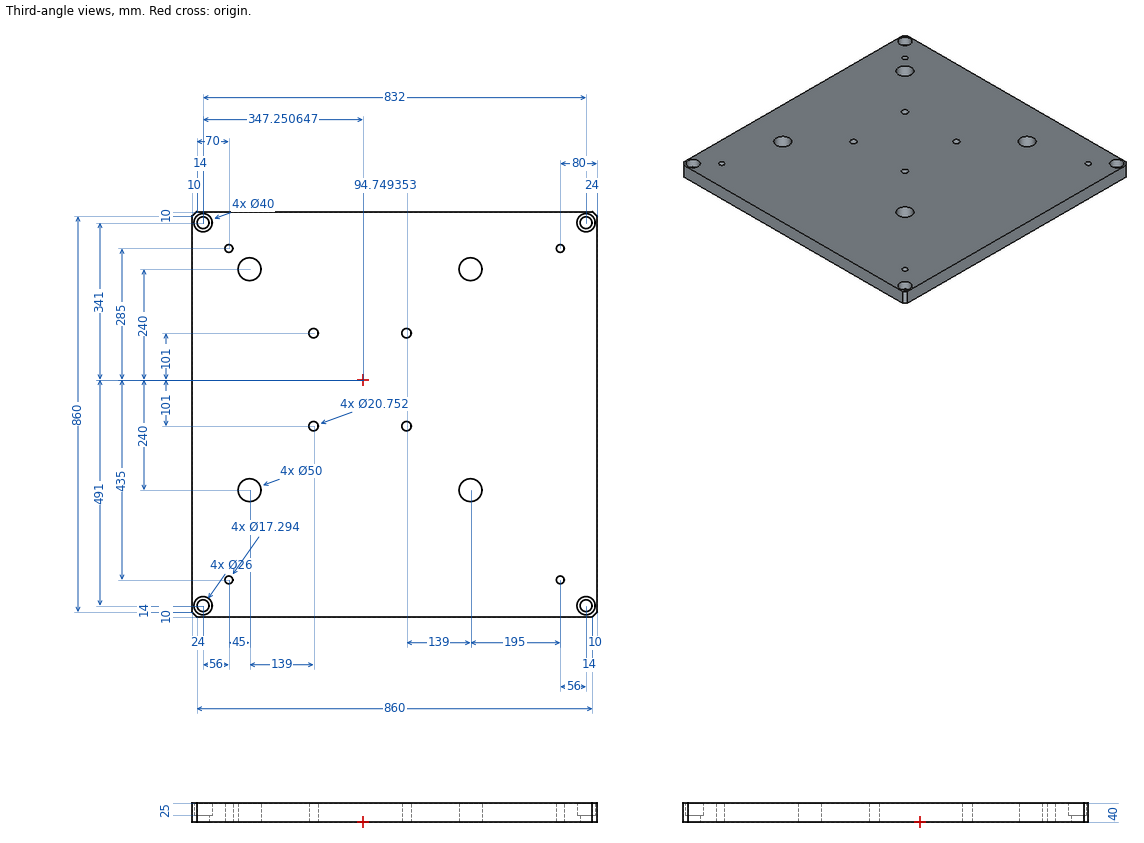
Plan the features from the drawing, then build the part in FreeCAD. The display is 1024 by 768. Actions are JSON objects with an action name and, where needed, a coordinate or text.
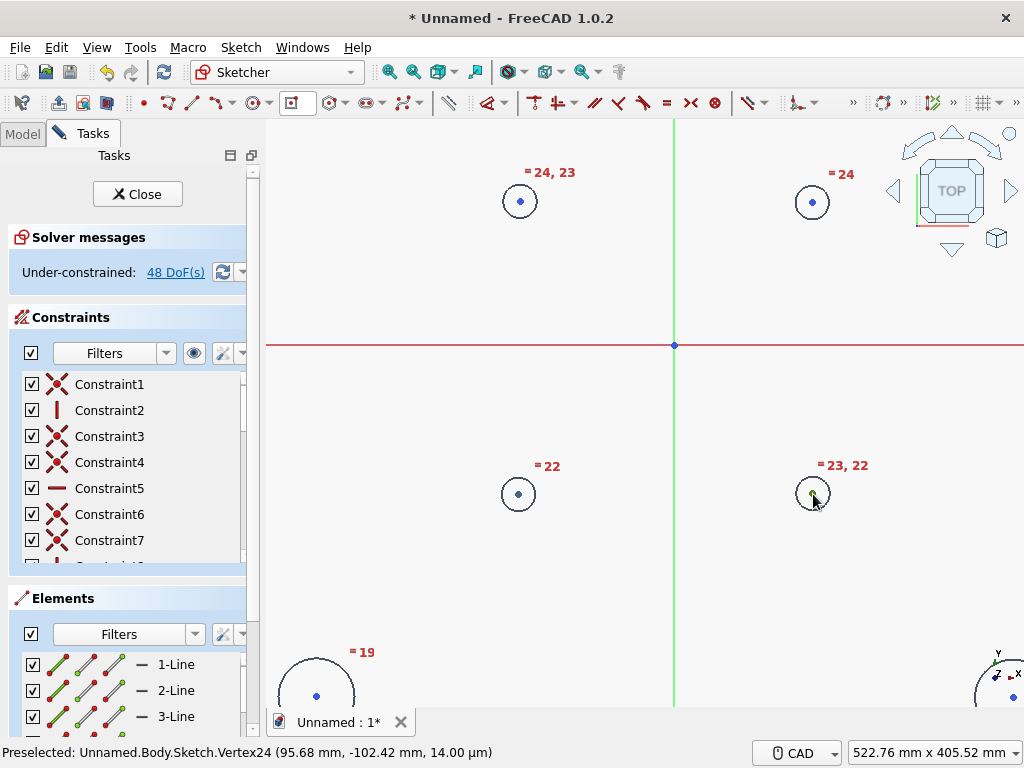
{"action": "key", "text": "h"}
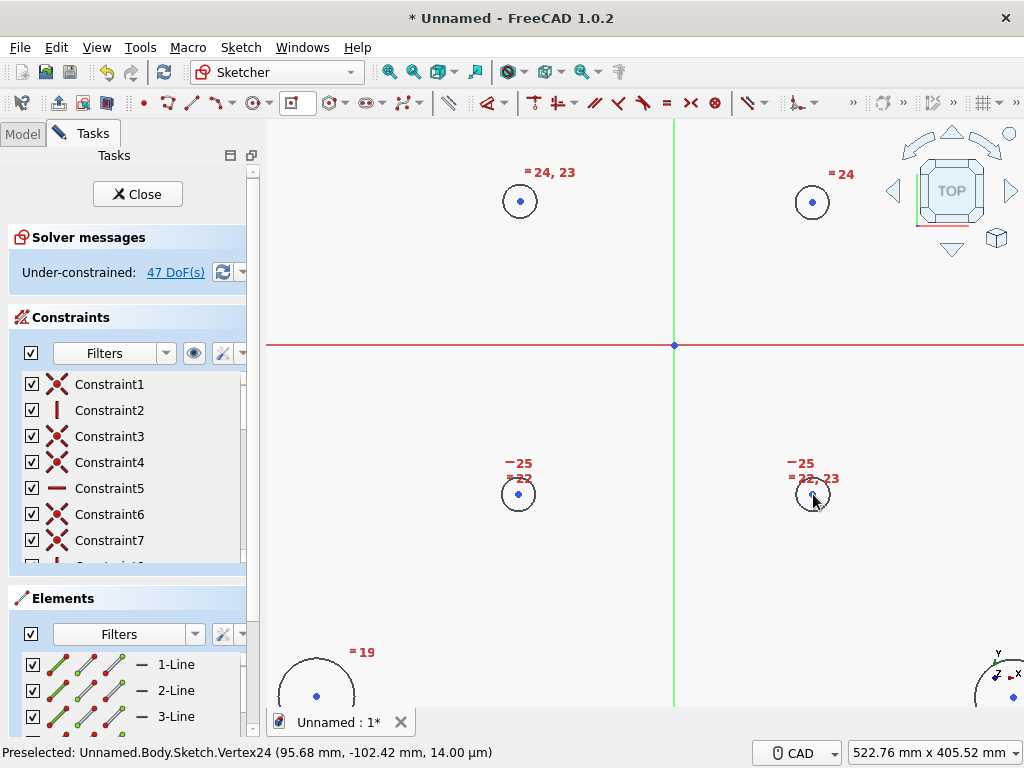
{"action": "left_click", "coordinate": [518, 494]}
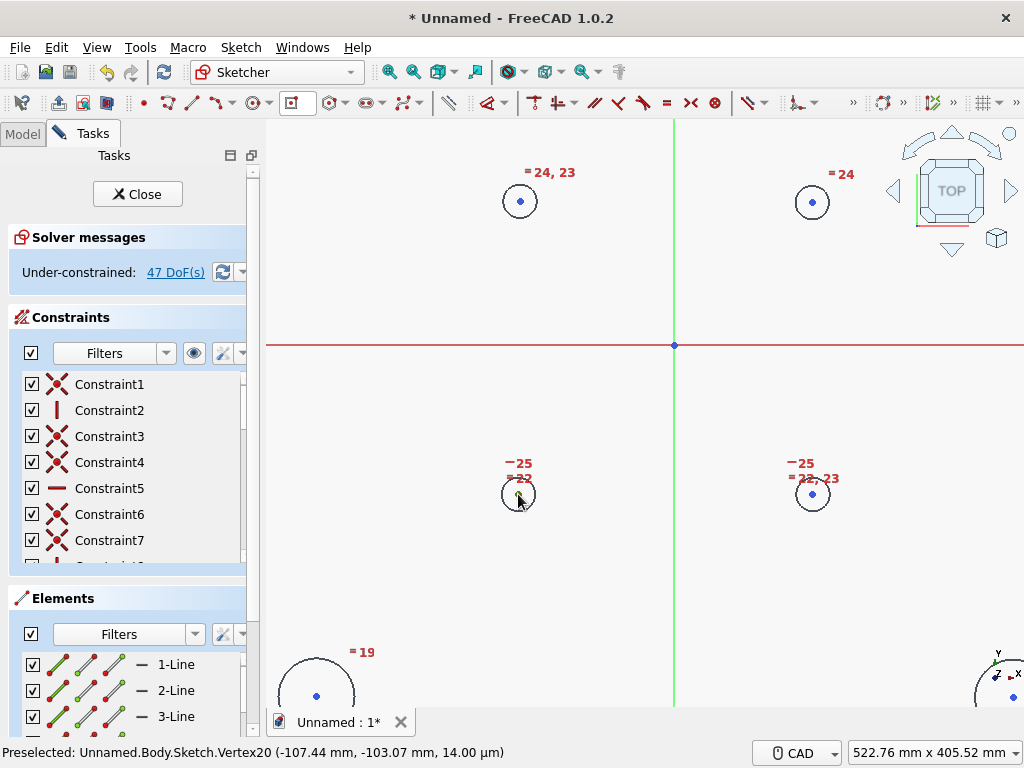
{"action": "left_click", "coordinate": [520, 201]}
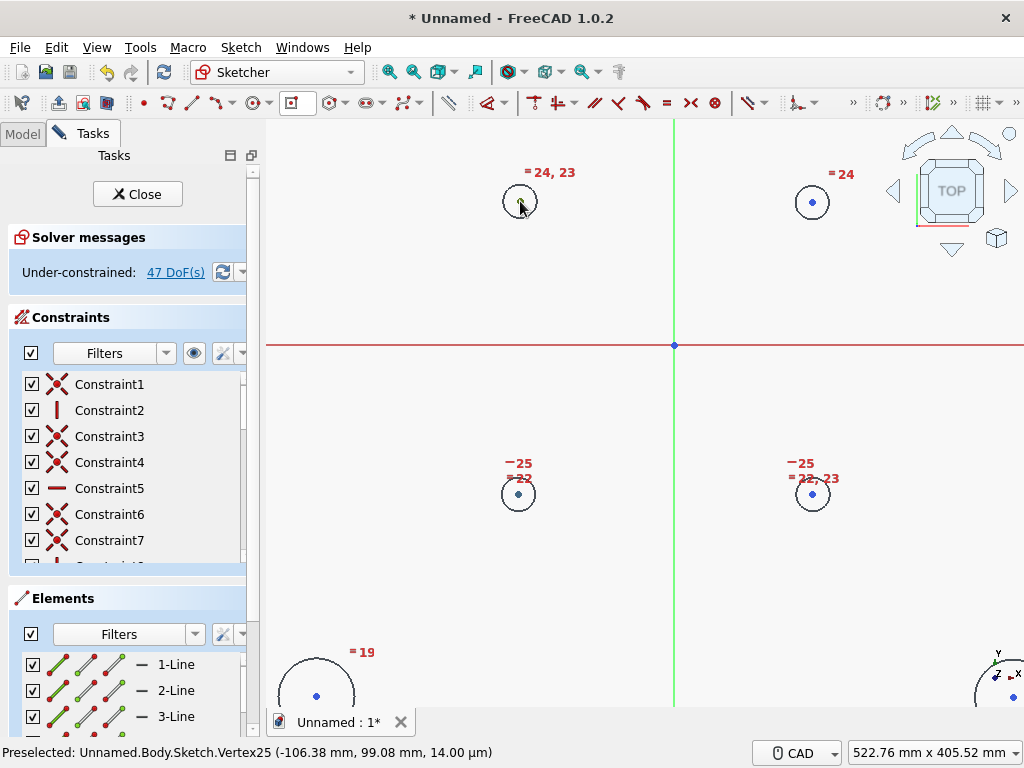
{"action": "key", "text": "v"}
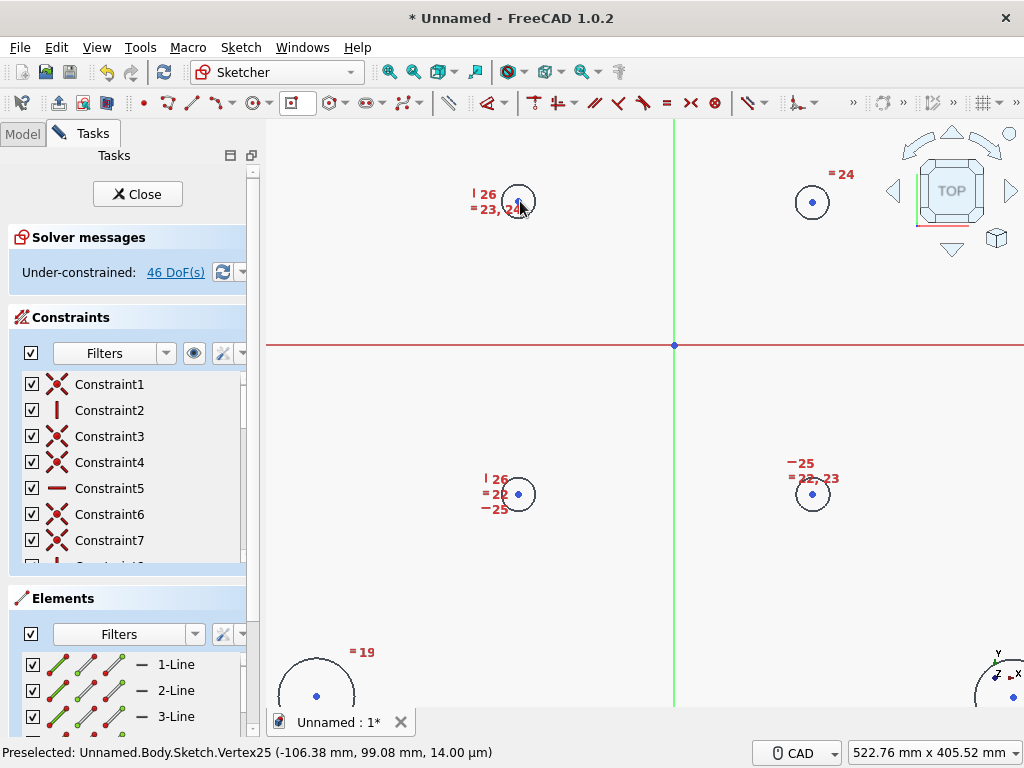
{"action": "left_click", "coordinate": [813, 494]}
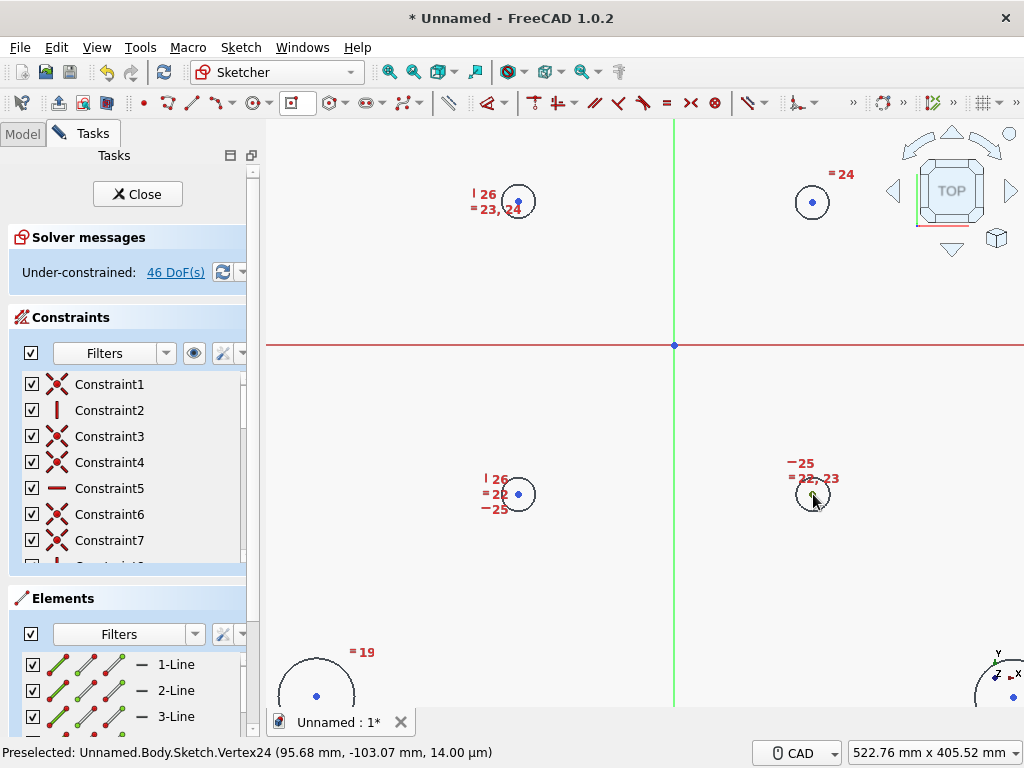
{"action": "left_click", "coordinate": [812, 203]}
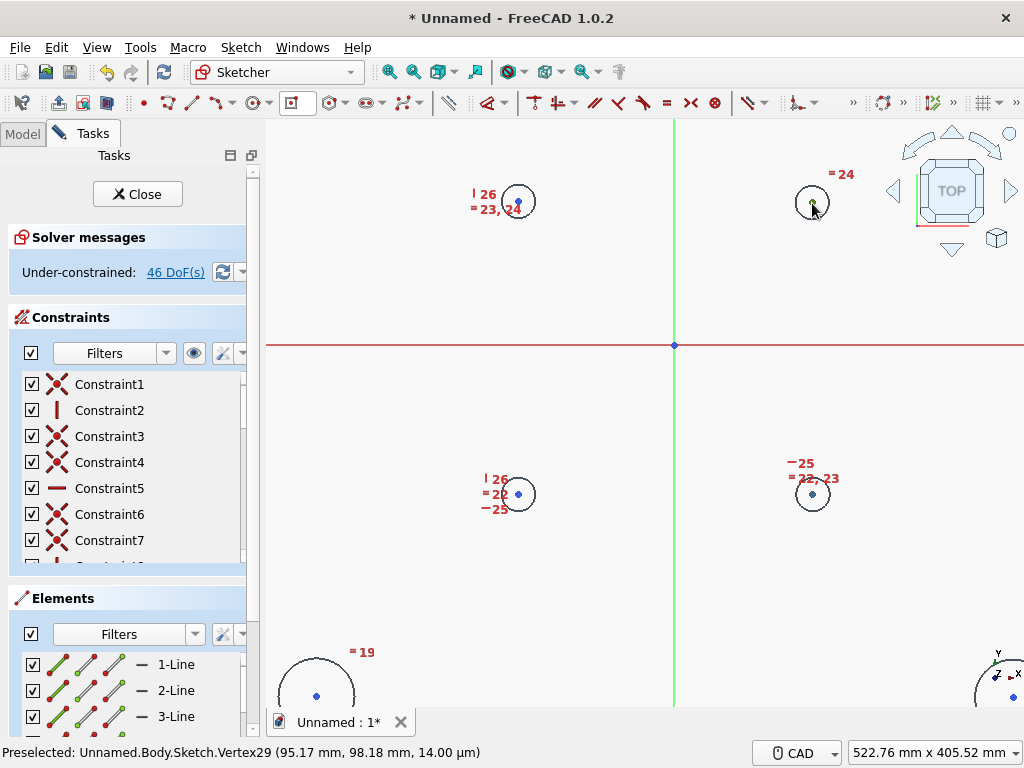
{"action": "key", "text": "v"}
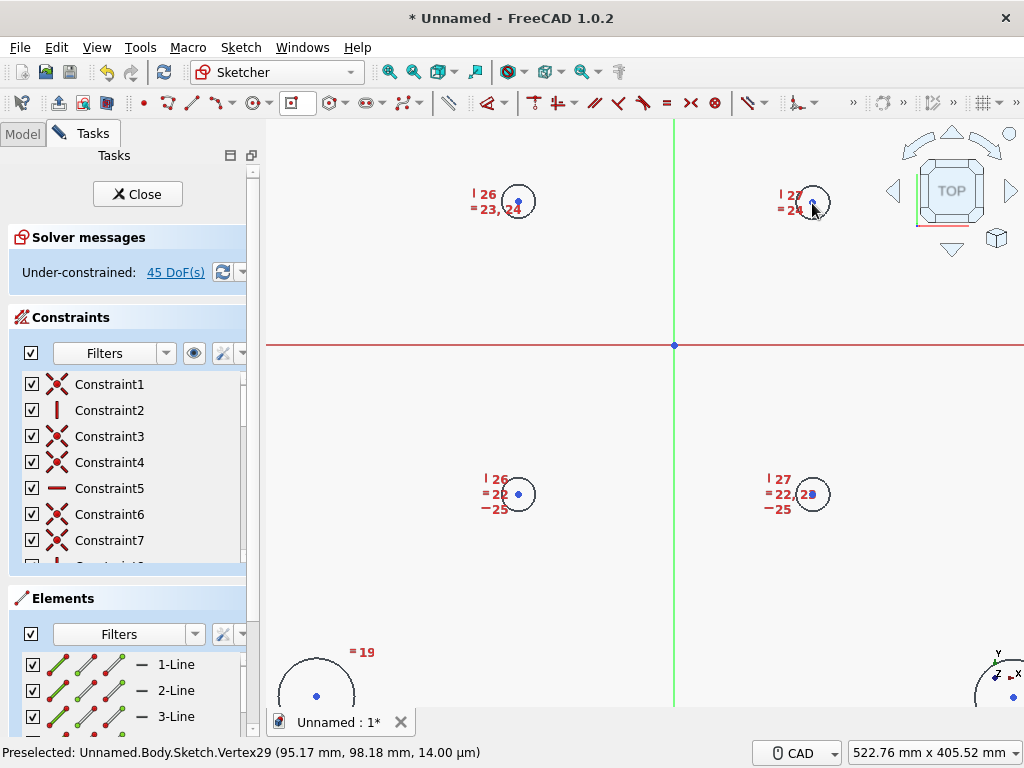
{"action": "scroll", "coordinate": [518, 201], "scroll_direction": "up", "scroll_amount": 4}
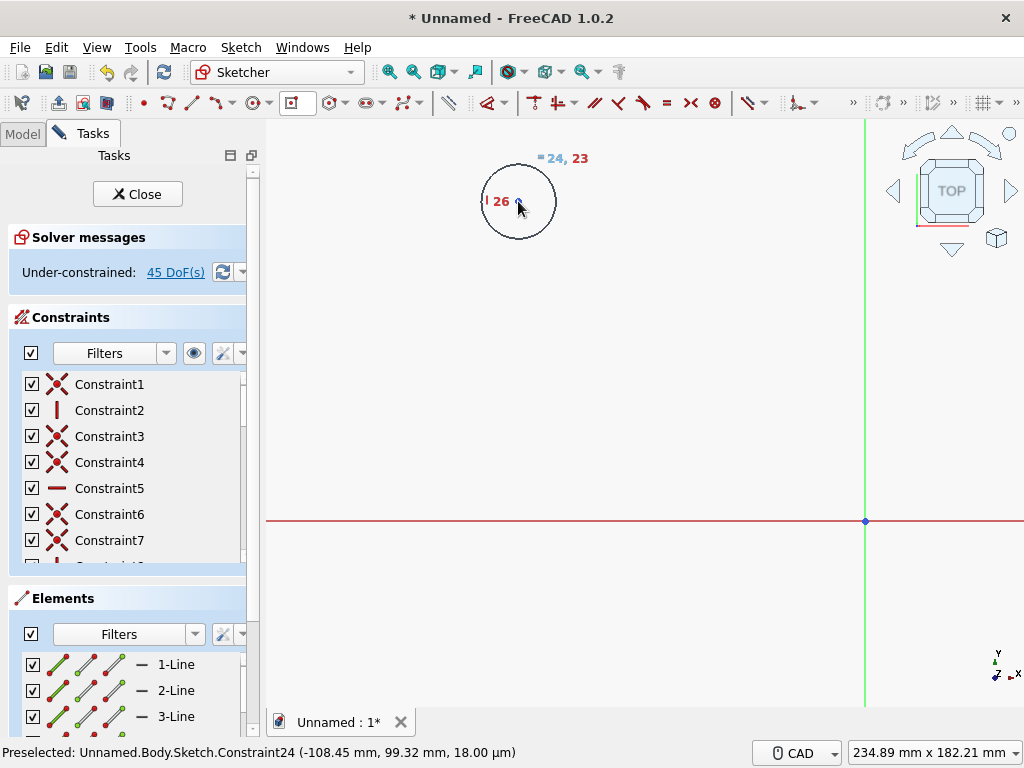
{"action": "left_click", "coordinate": [519, 202]}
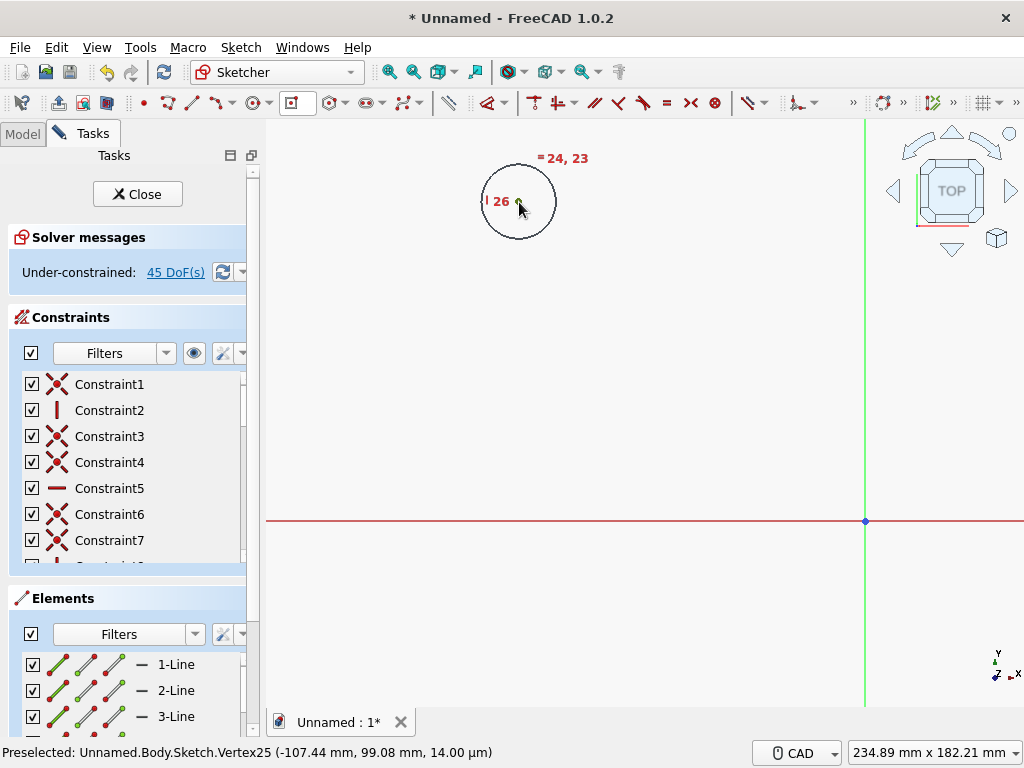
{"action": "scroll", "coordinate": [497, 358], "scroll_direction": "down", "scroll_amount": 10}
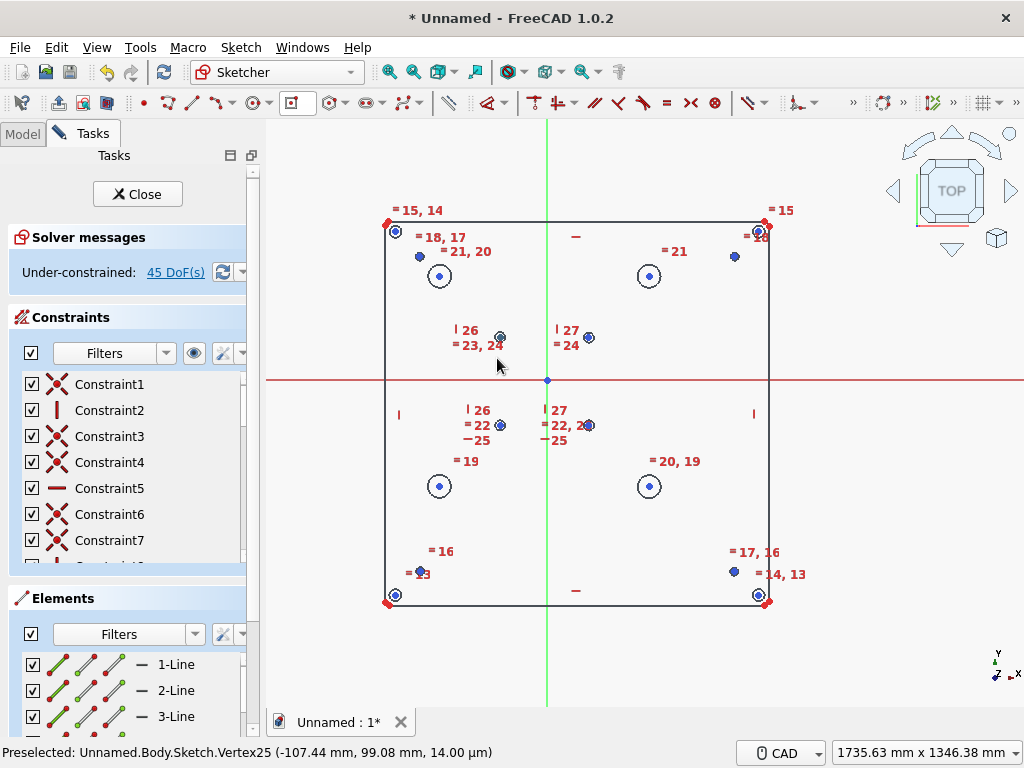
{"action": "left_click", "coordinate": [589, 338]}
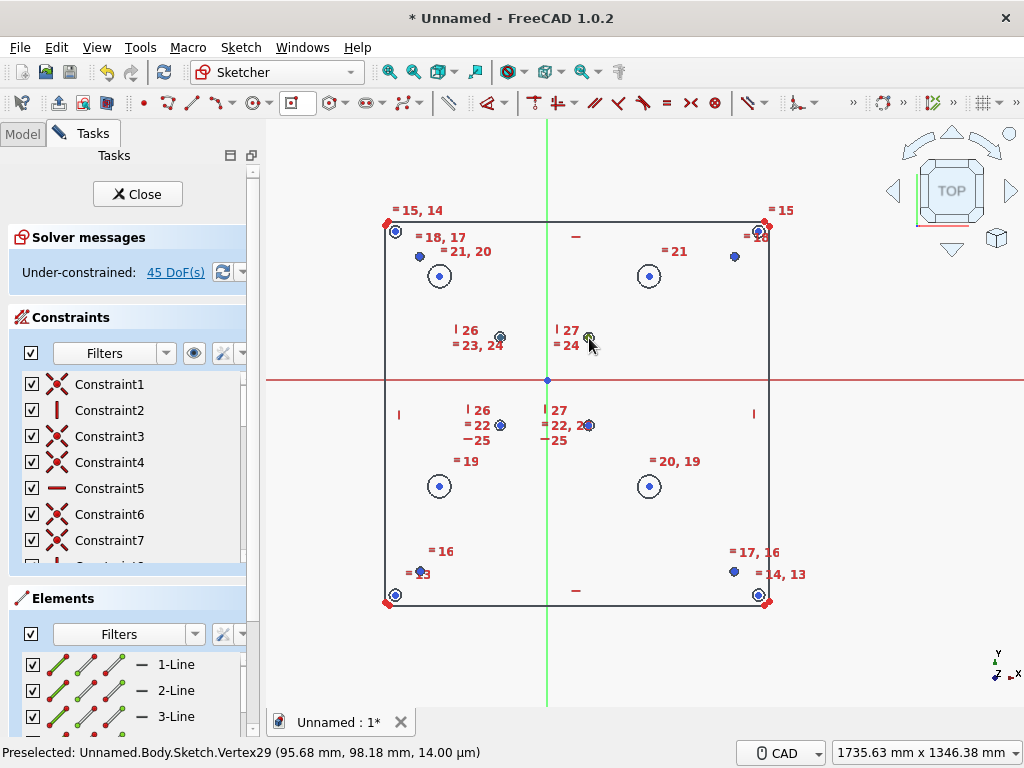
{"action": "left_click", "coordinate": [576, 104]}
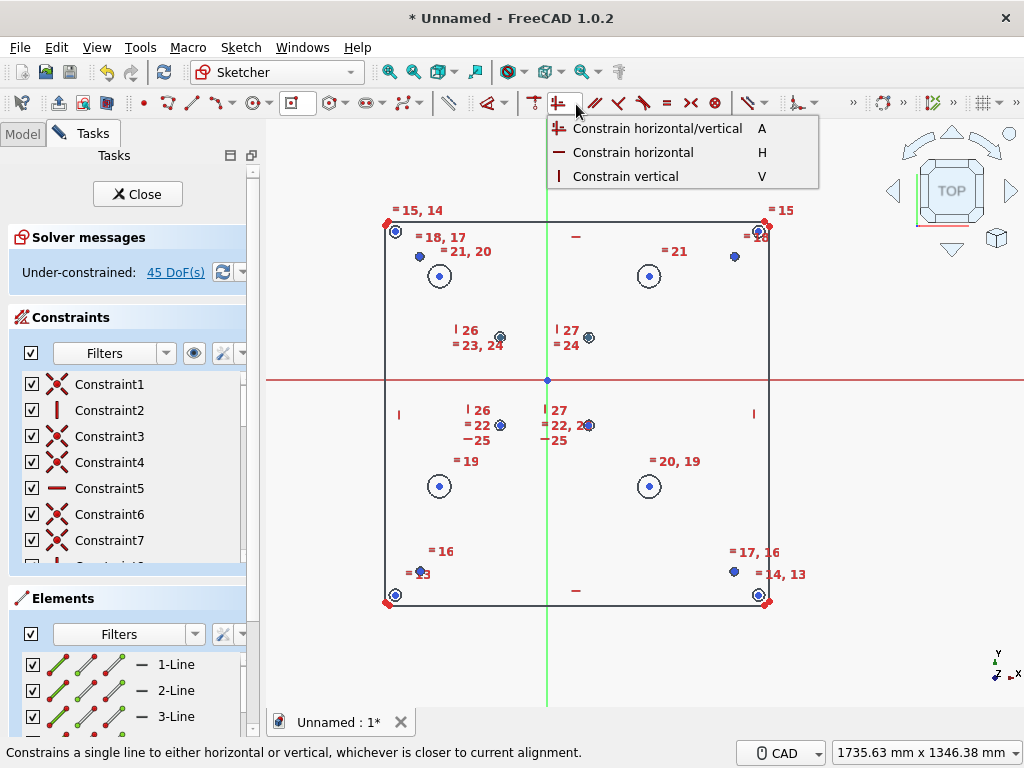
{"action": "left_click", "coordinate": [683, 152]}